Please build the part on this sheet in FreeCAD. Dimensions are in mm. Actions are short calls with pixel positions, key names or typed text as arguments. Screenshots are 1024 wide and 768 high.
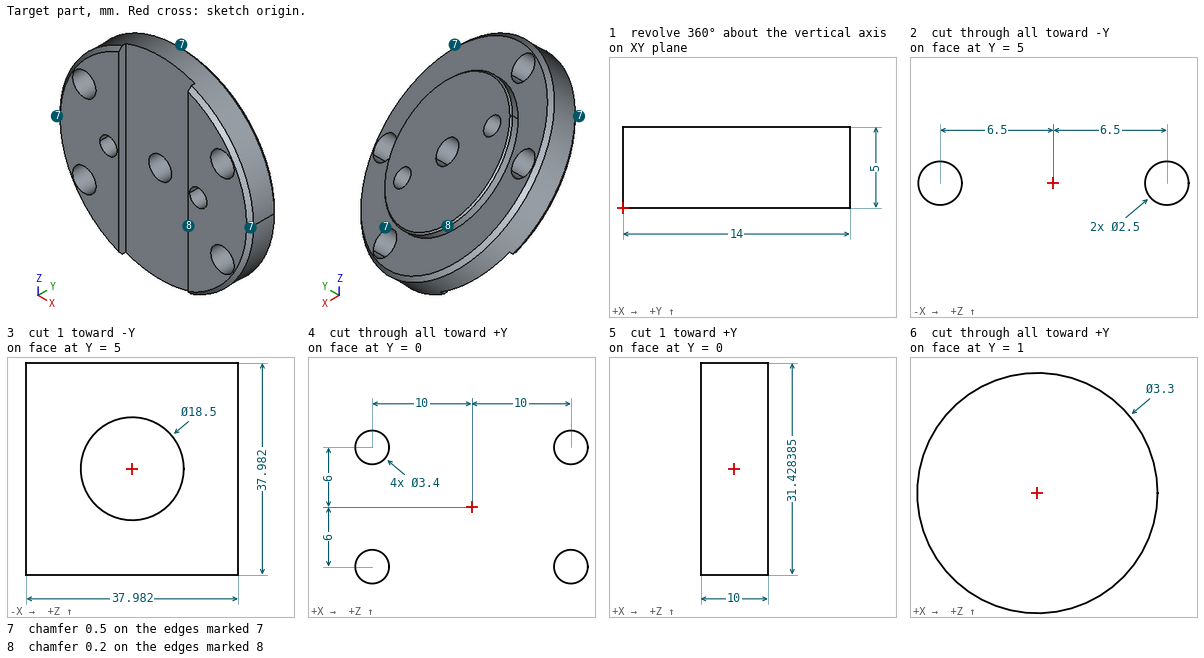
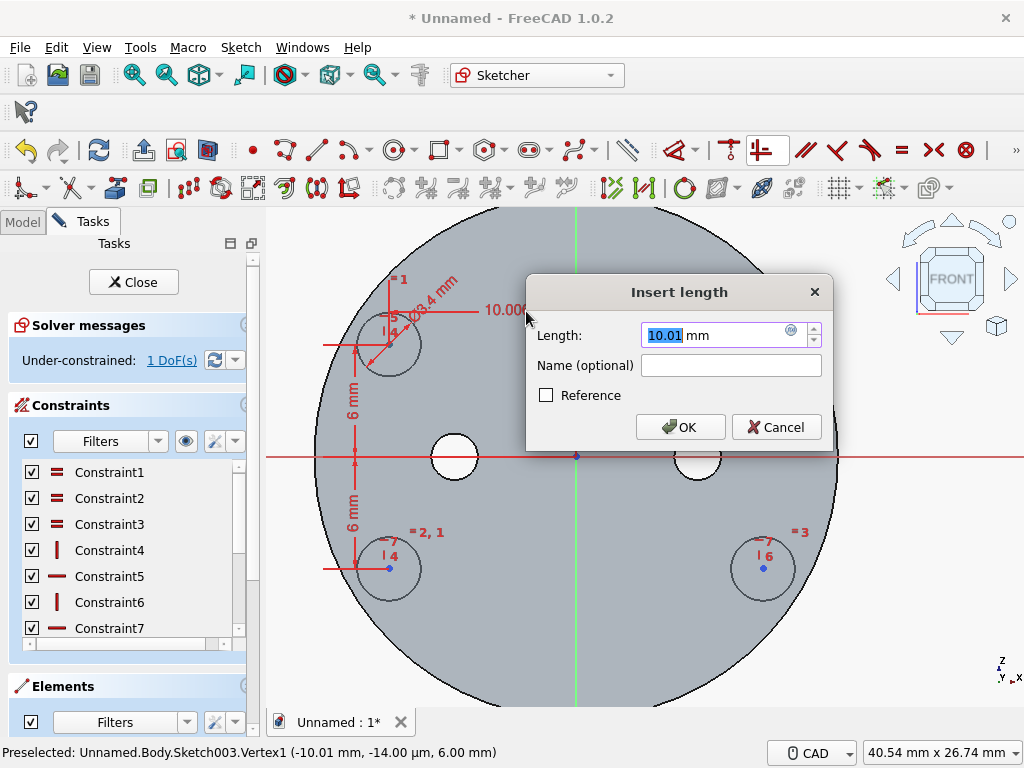
text(10)
key(Return)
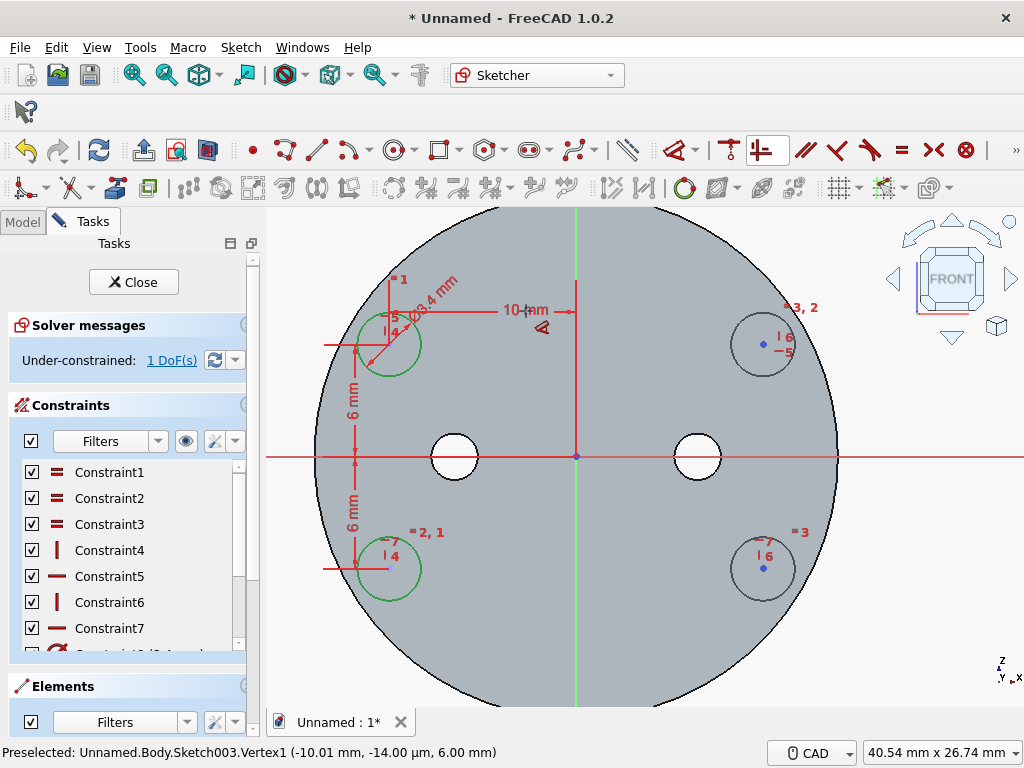
click(763, 345)
click(670, 311)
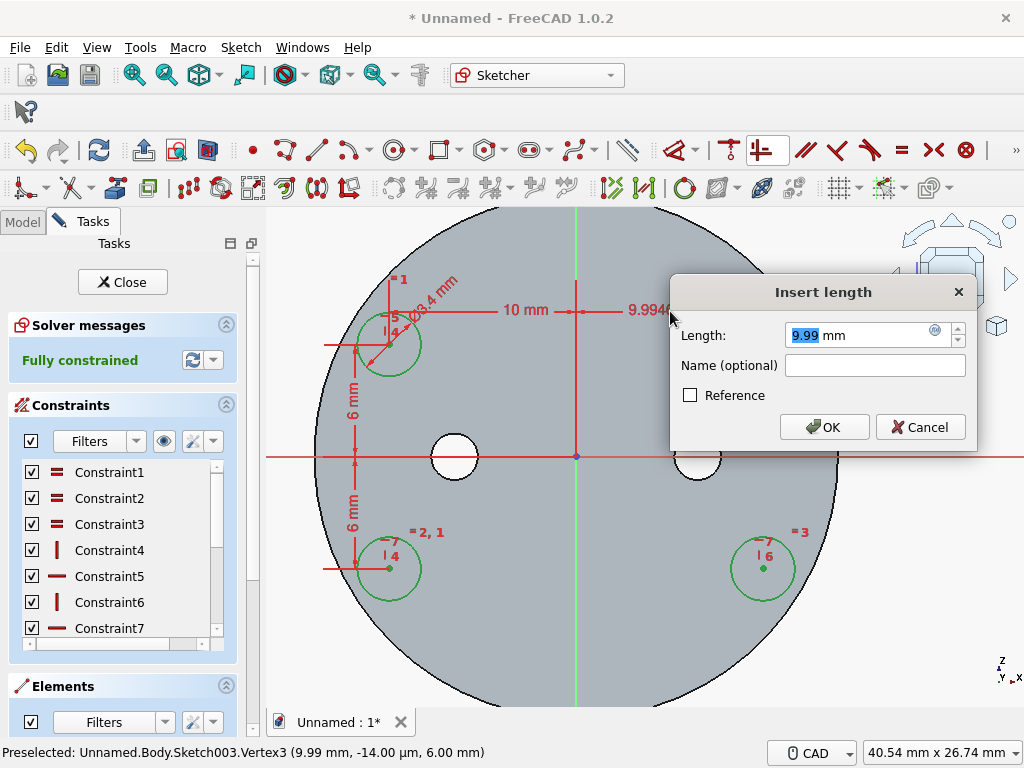
text(10)
key(Return)
key(Escape)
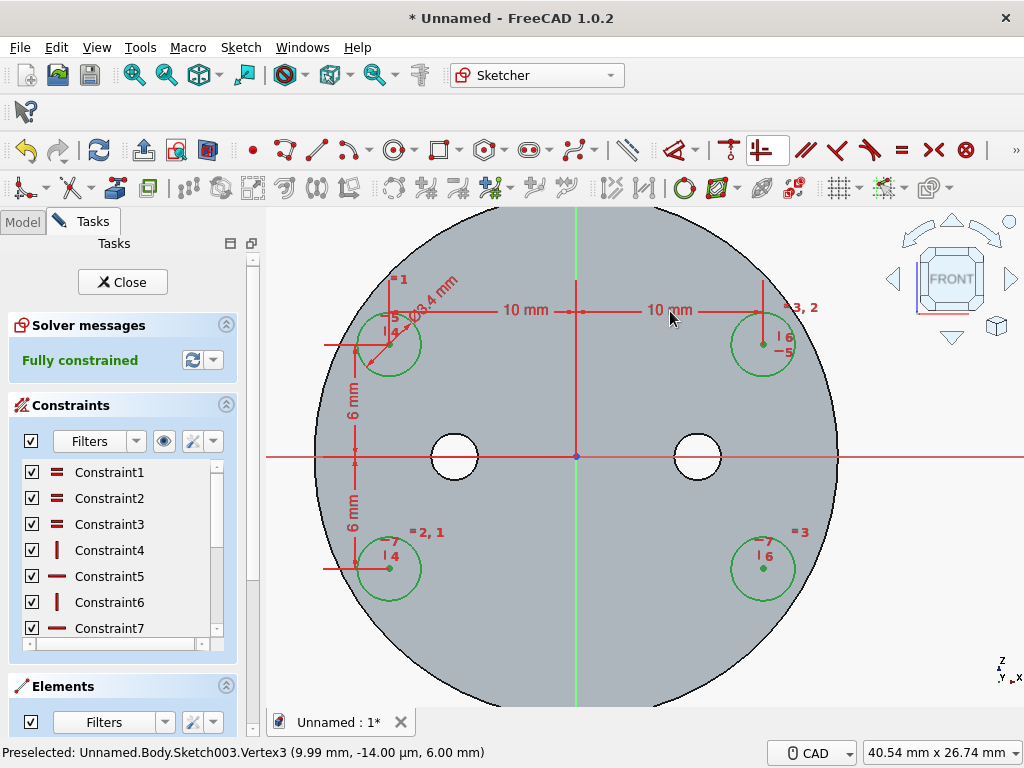
click(123, 282)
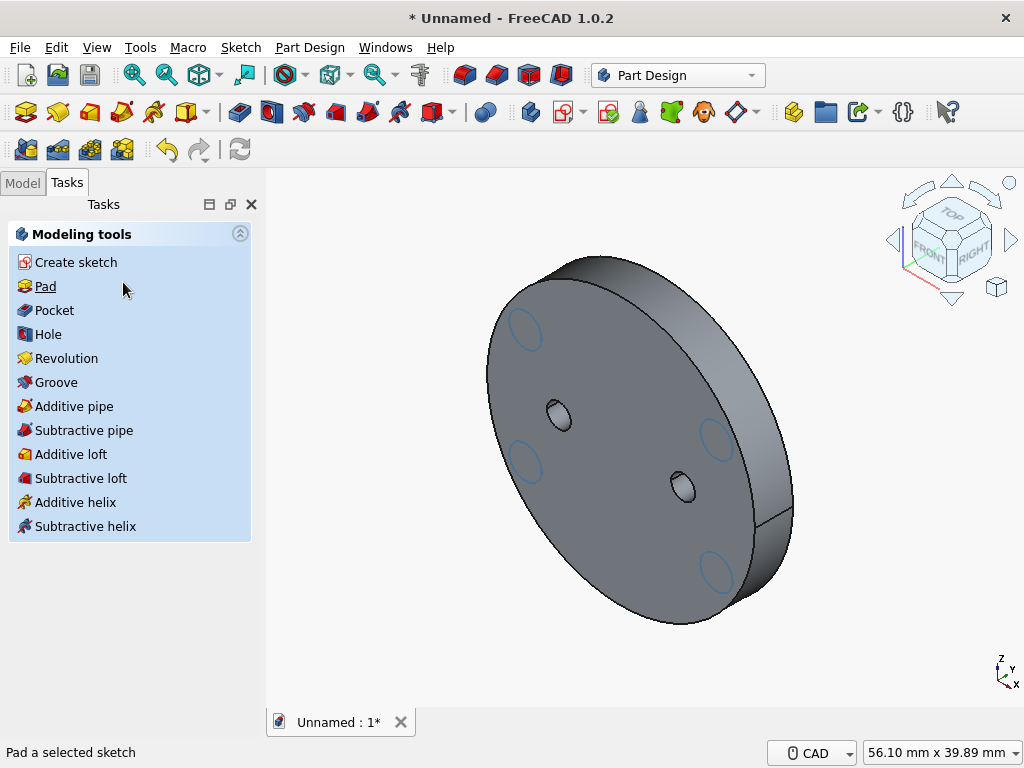
click(240, 112)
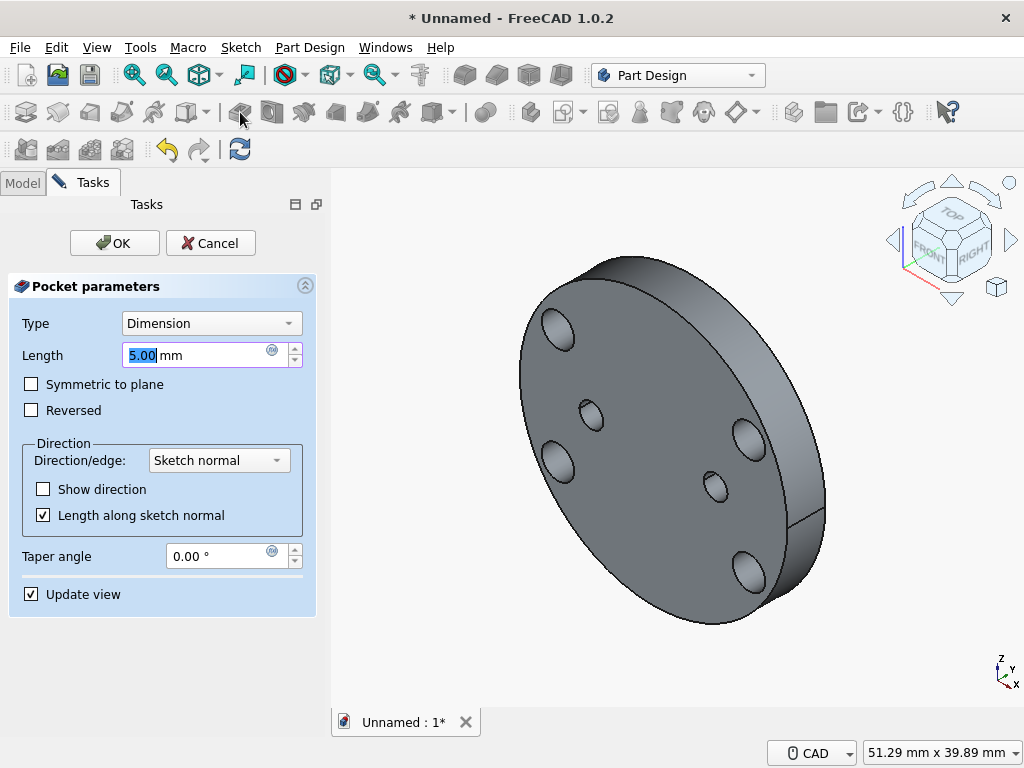
click(212, 324)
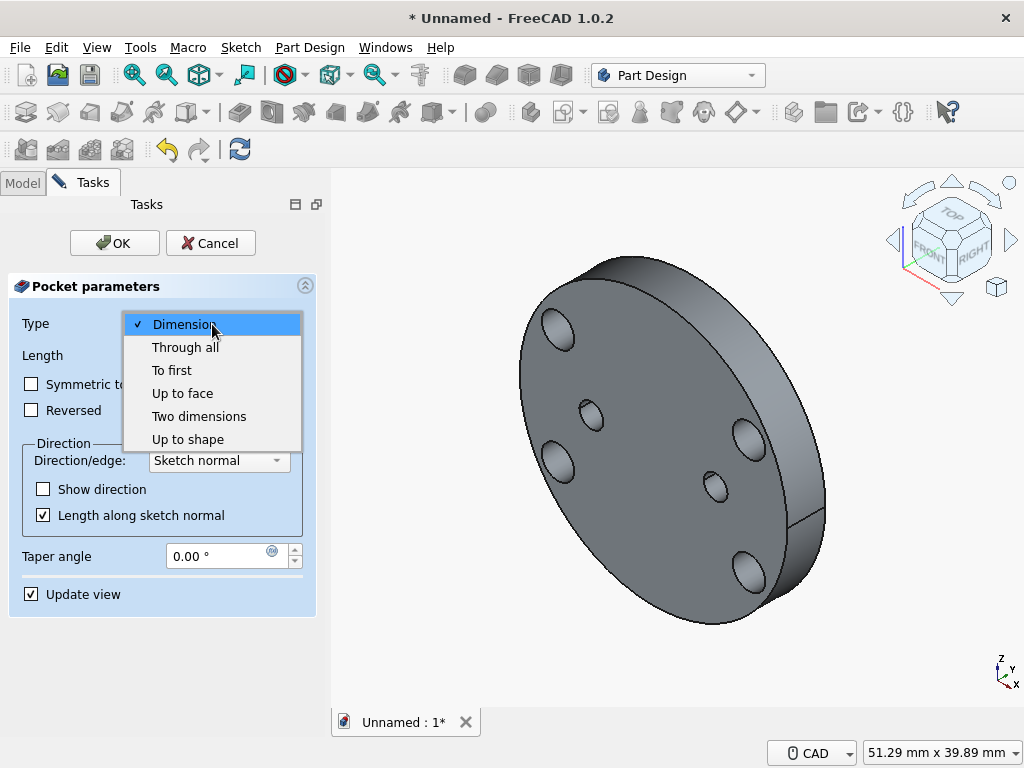
click(212, 348)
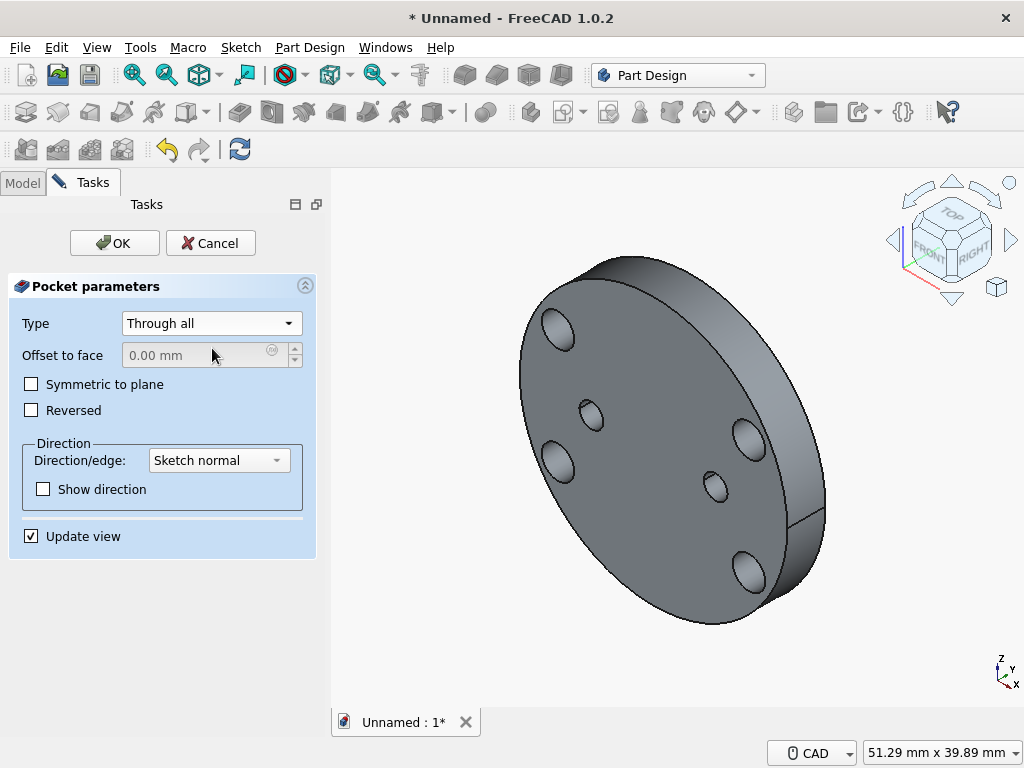
click(115, 243)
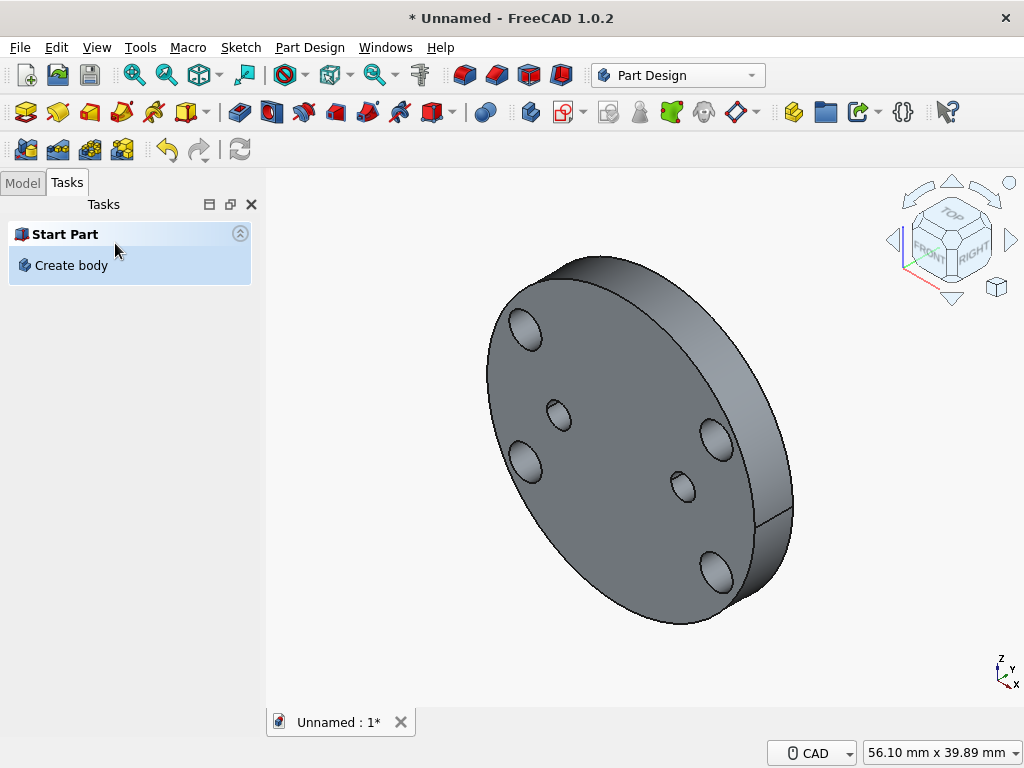
click(621, 494)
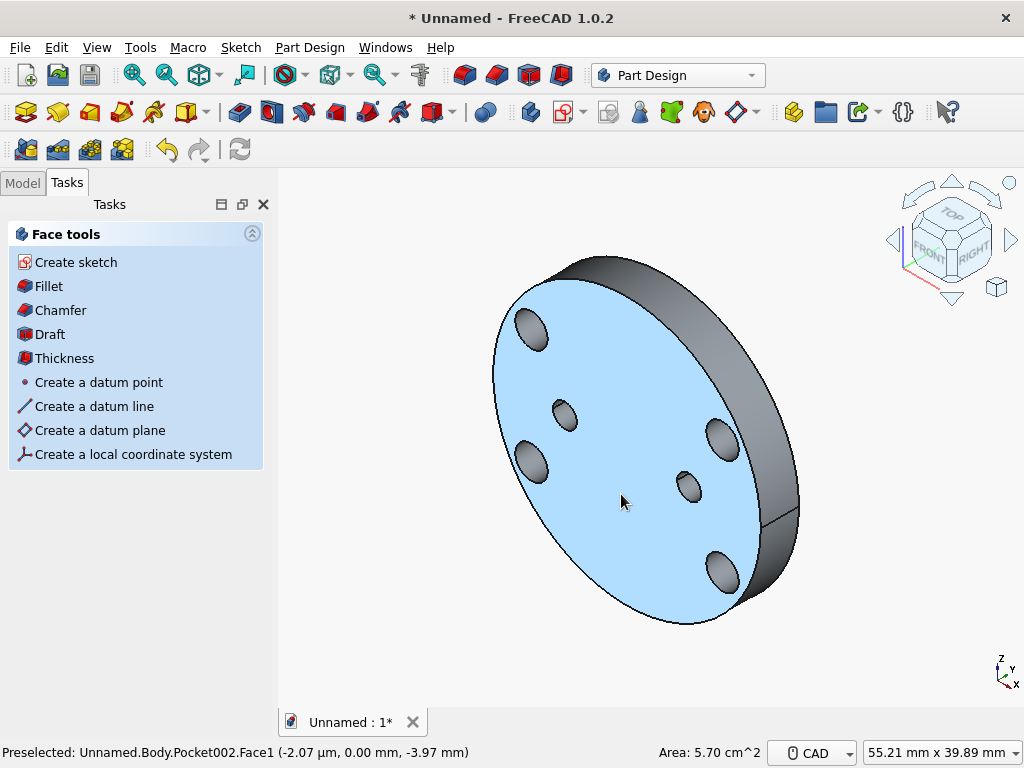
click(564, 112)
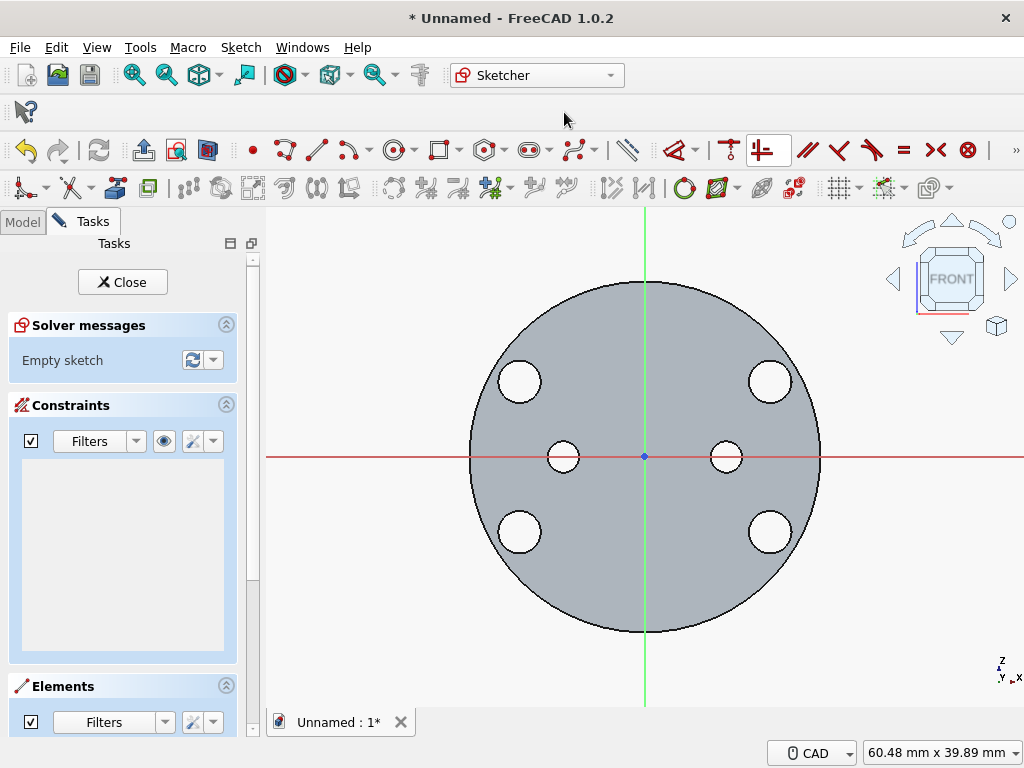
click(462, 150)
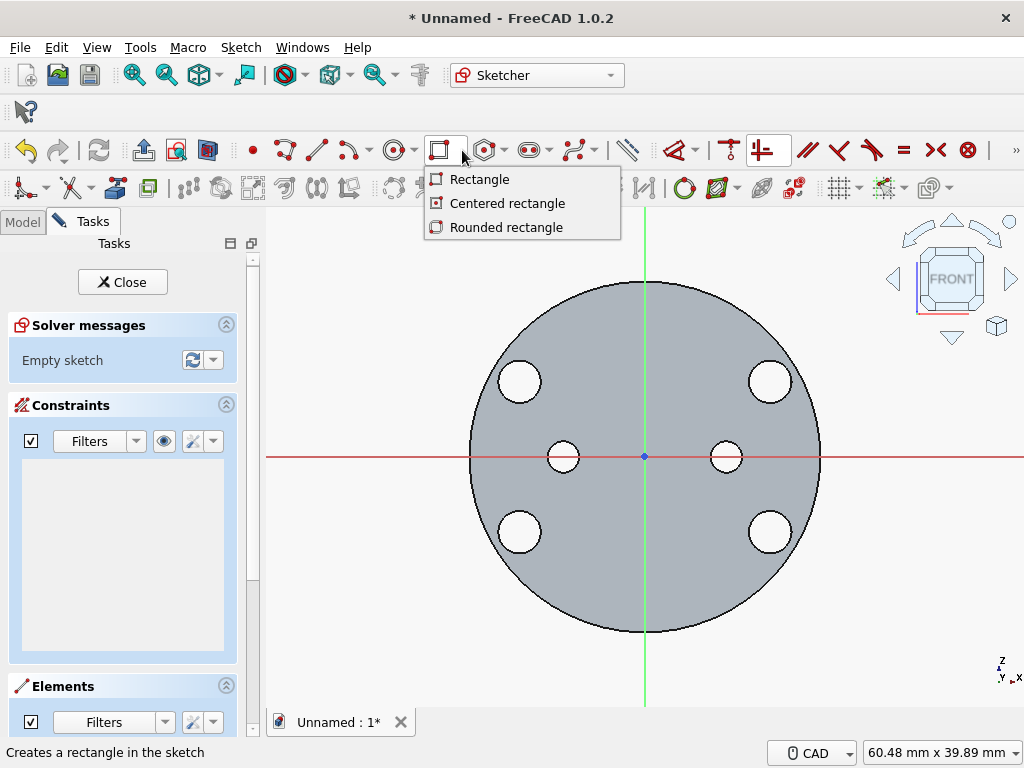
click(522, 203)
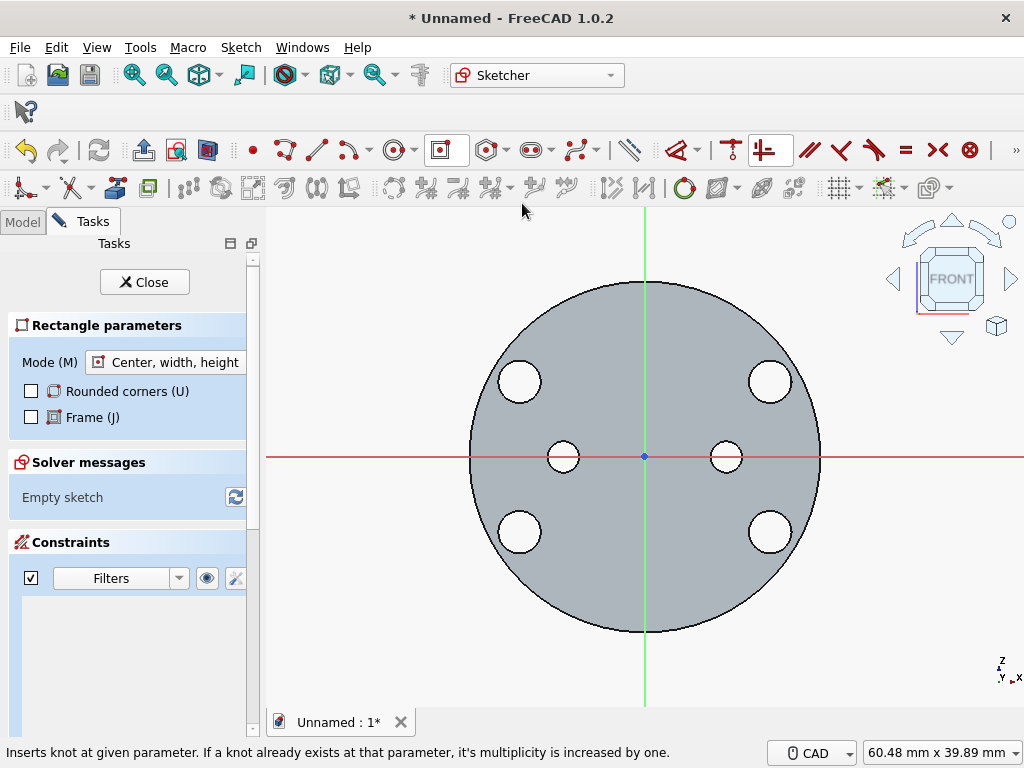
click(645, 457)
click(708, 260)
key(Escape)